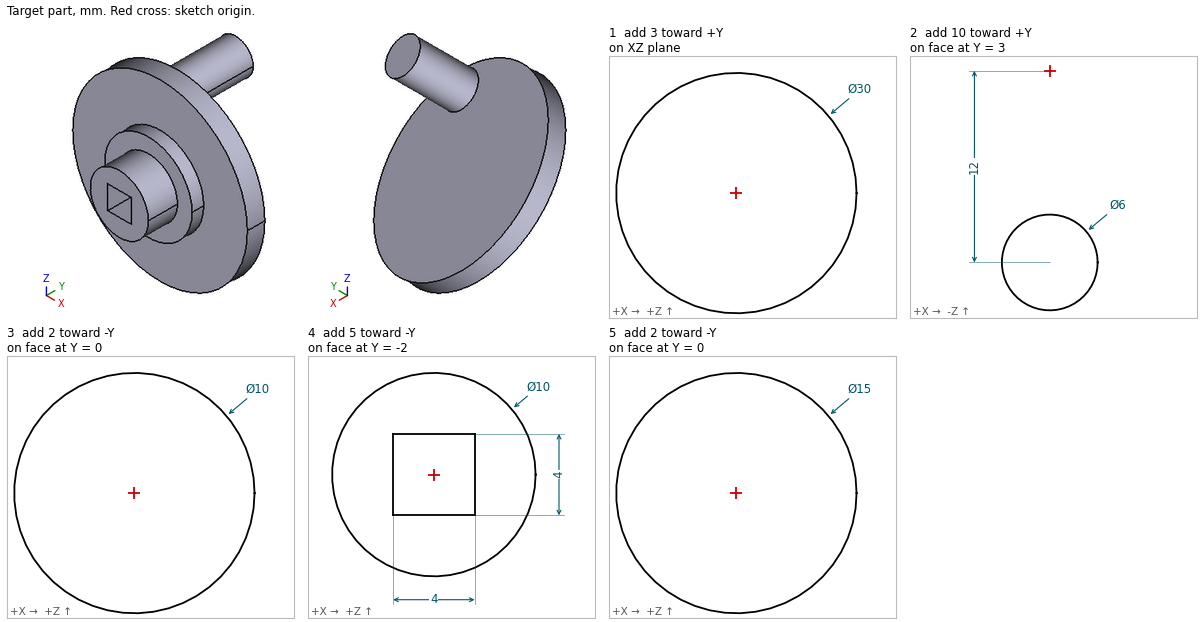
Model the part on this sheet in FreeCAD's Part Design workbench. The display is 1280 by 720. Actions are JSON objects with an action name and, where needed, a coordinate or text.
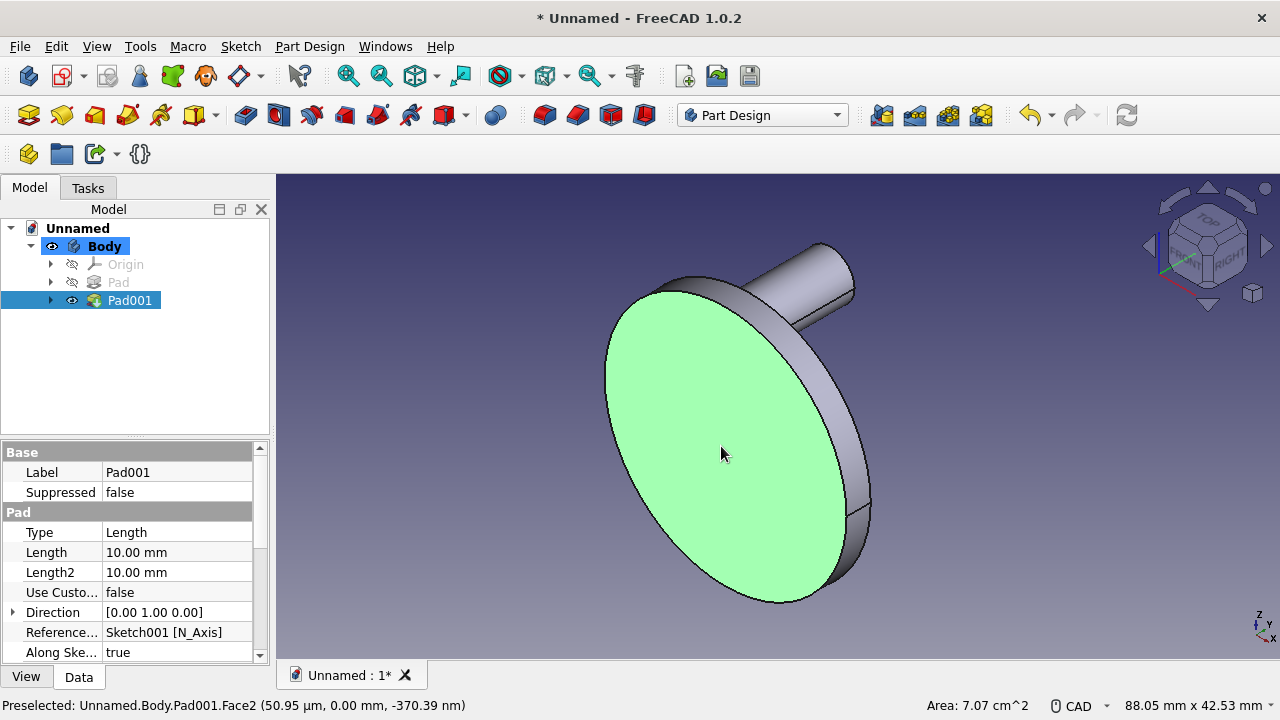
{"action": "left_click", "coordinate": [62, 76]}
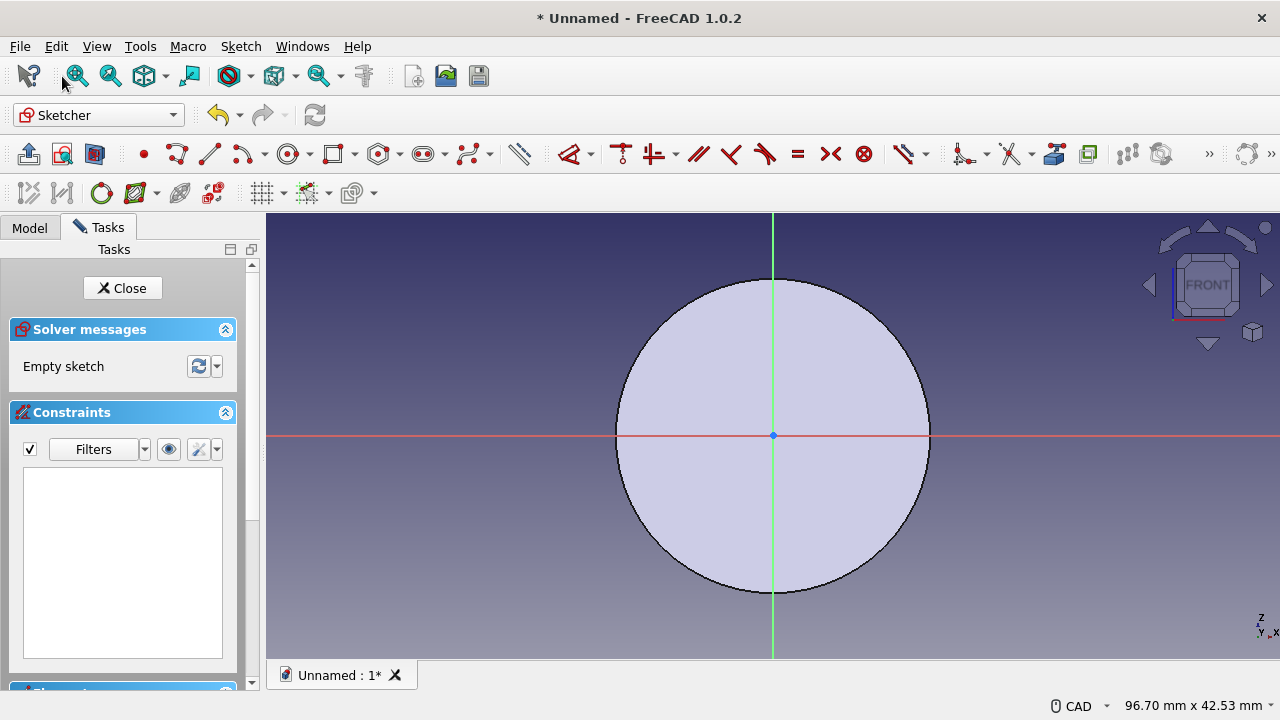
{"action": "scroll", "coordinate": [813, 436], "scroll_direction": "up", "scroll_amount": 5}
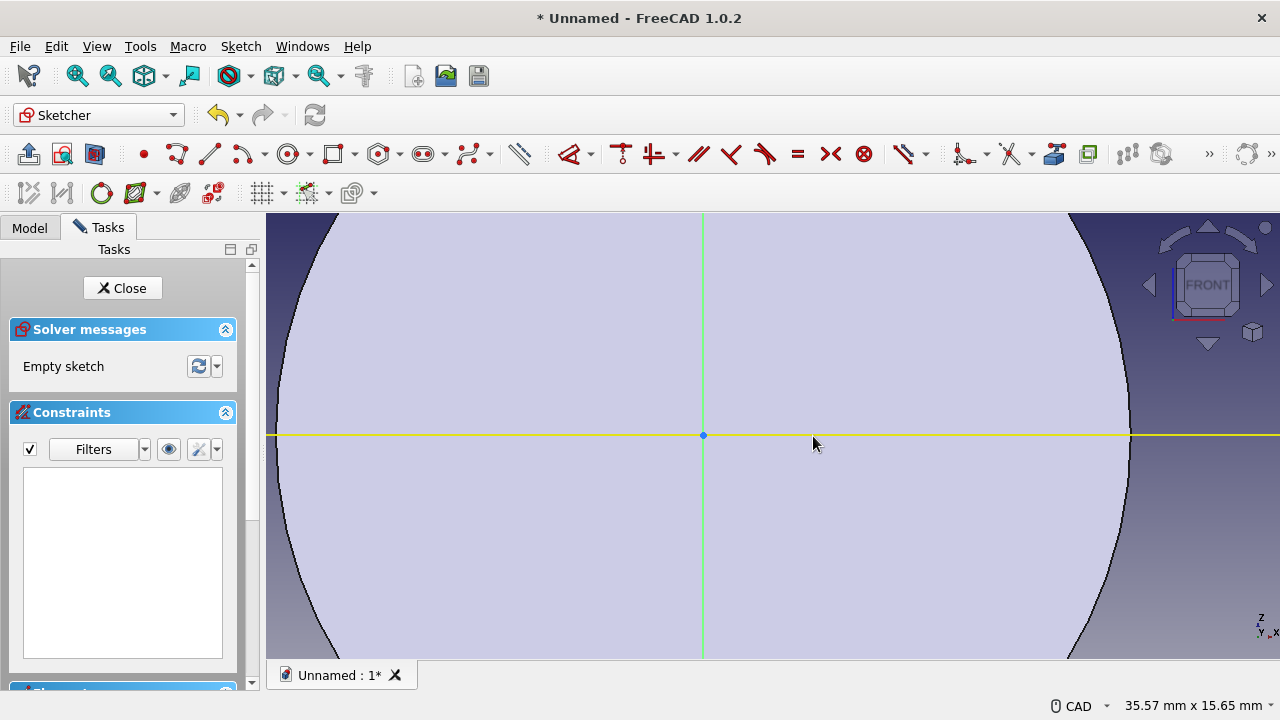
{"action": "left_click", "coordinate": [288, 154]}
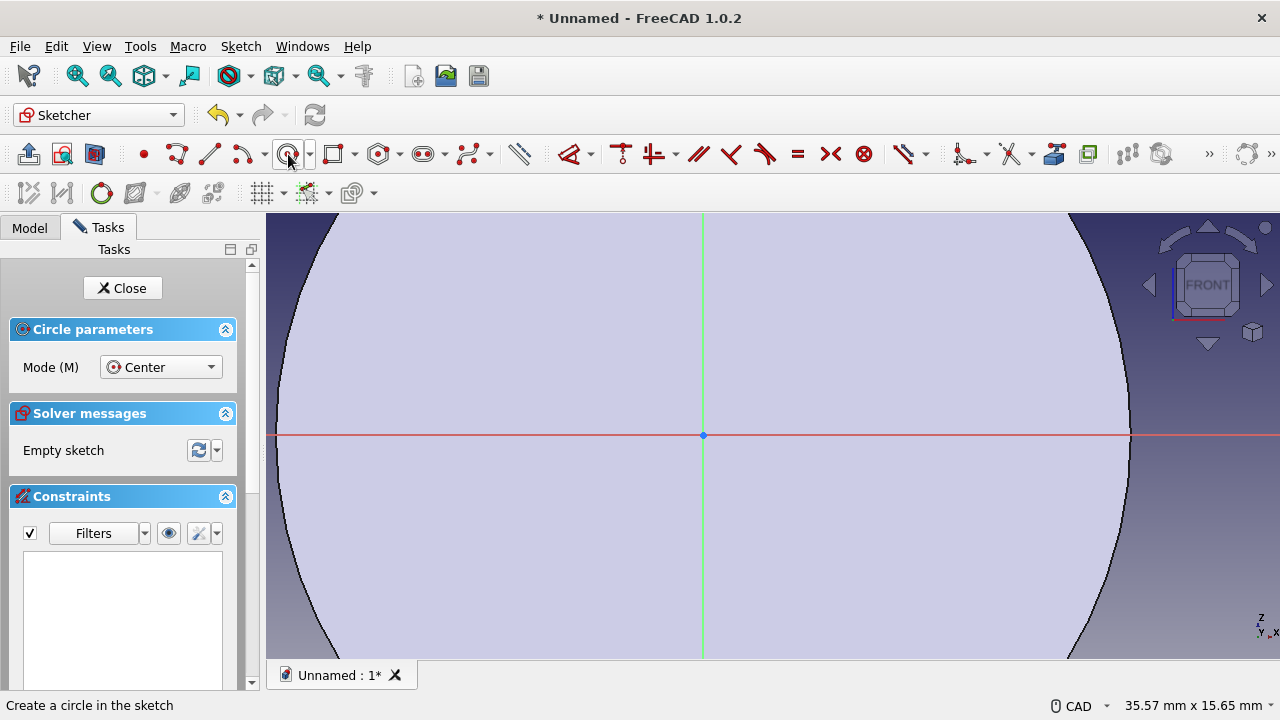
{"action": "left_click", "coordinate": [703, 435]}
{"action": "left_click", "coordinate": [804, 334]}
{"action": "key", "text": "Escape"}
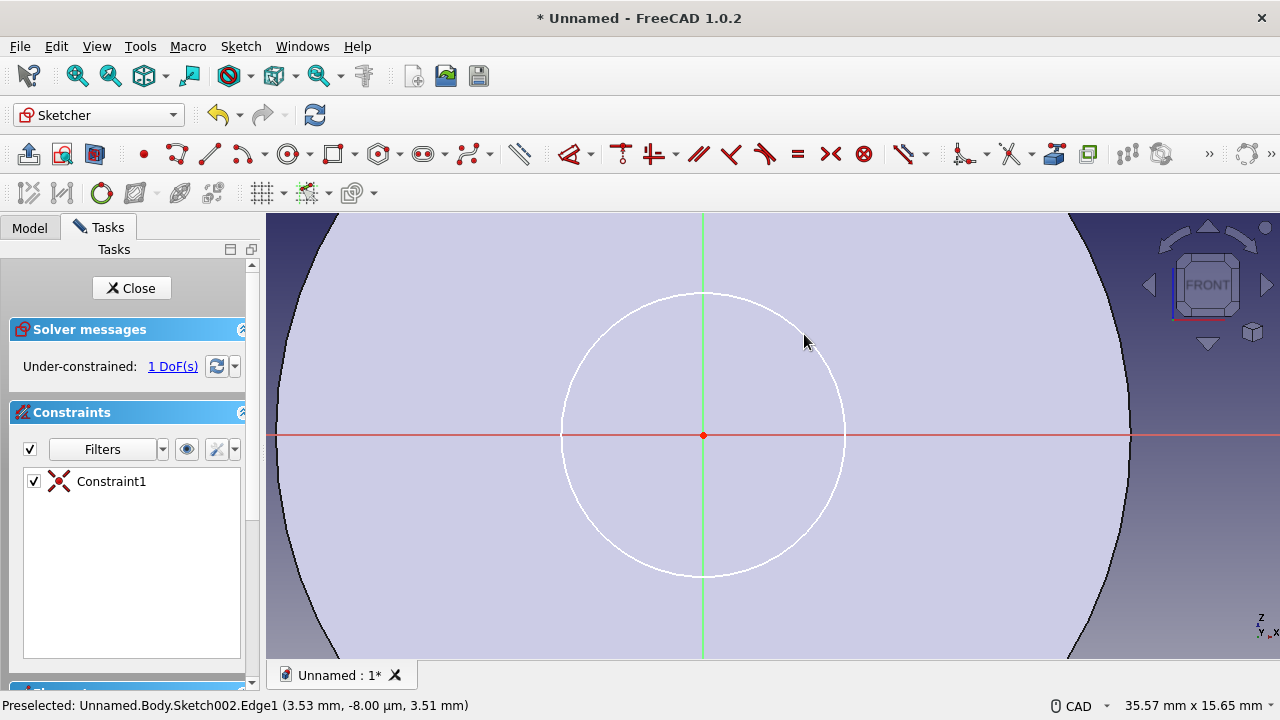
{"action": "left_click", "coordinate": [568, 154]}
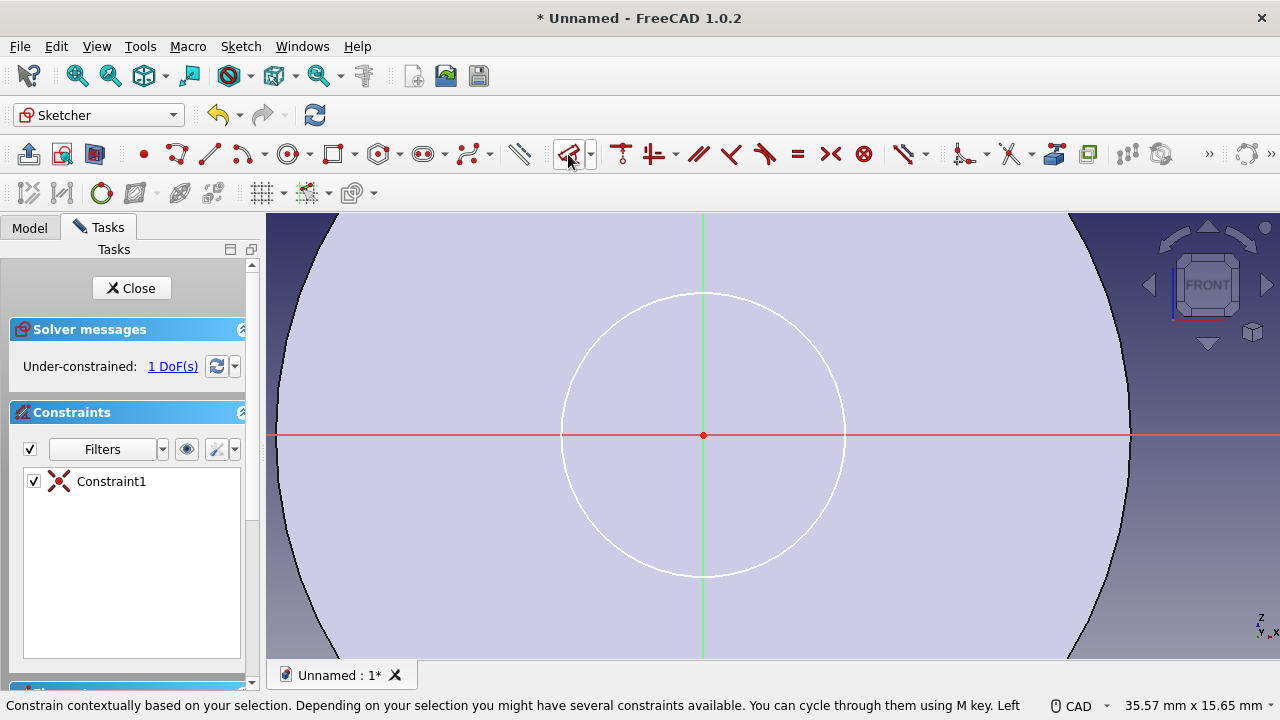
{"action": "left_click", "coordinate": [803, 334]}
{"action": "left_click", "coordinate": [825, 311]}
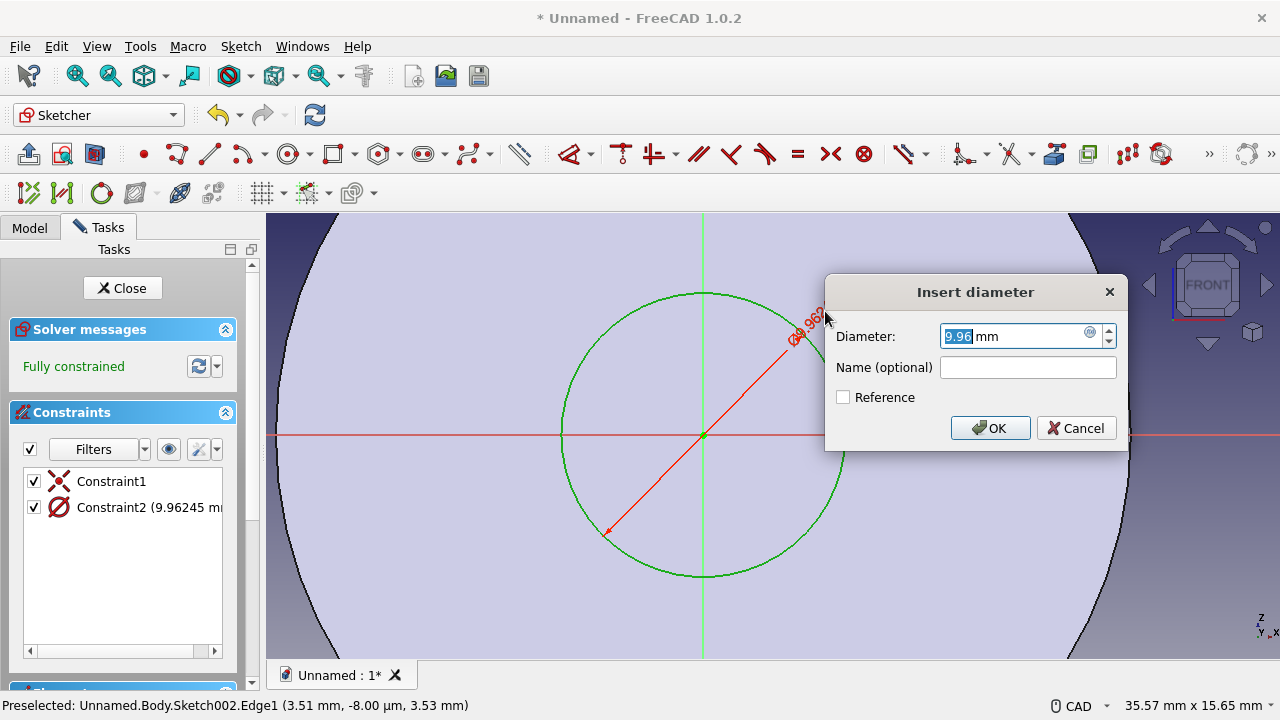
{"action": "type", "text": "10"}
{"action": "key", "text": "Return"}
{"action": "key", "text": "Escape"}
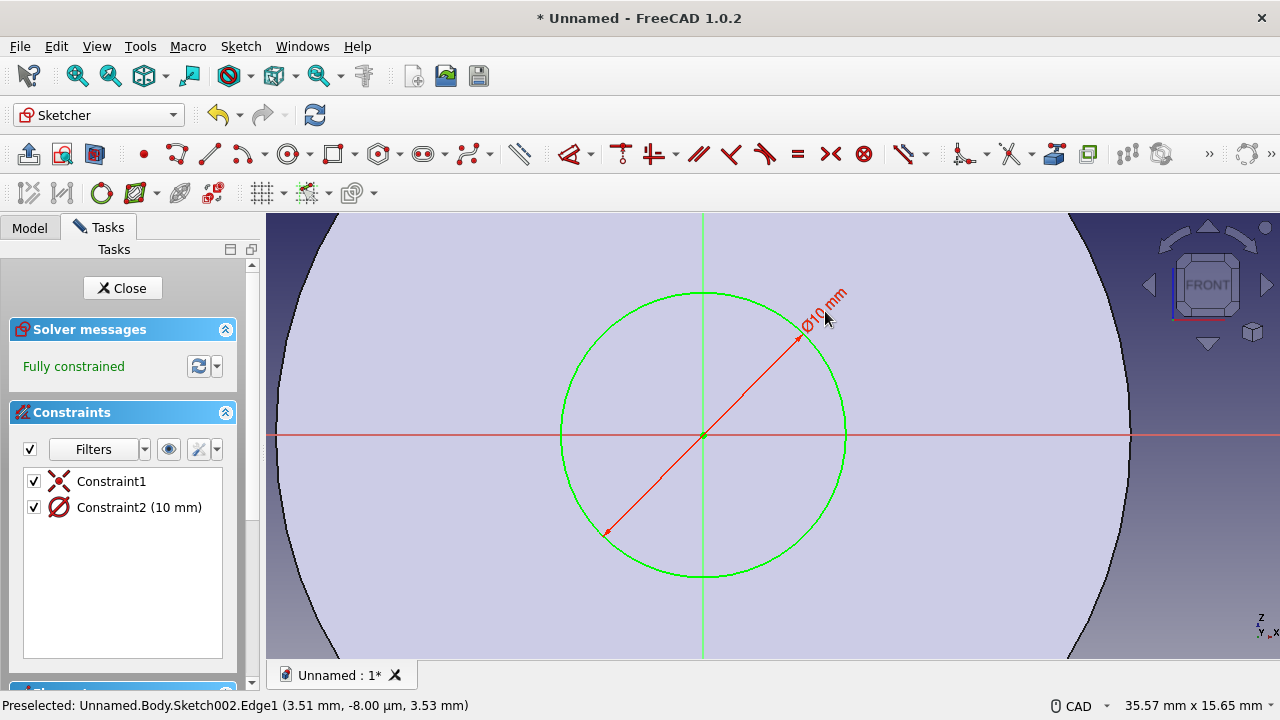
{"action": "left_click", "coordinate": [123, 288]}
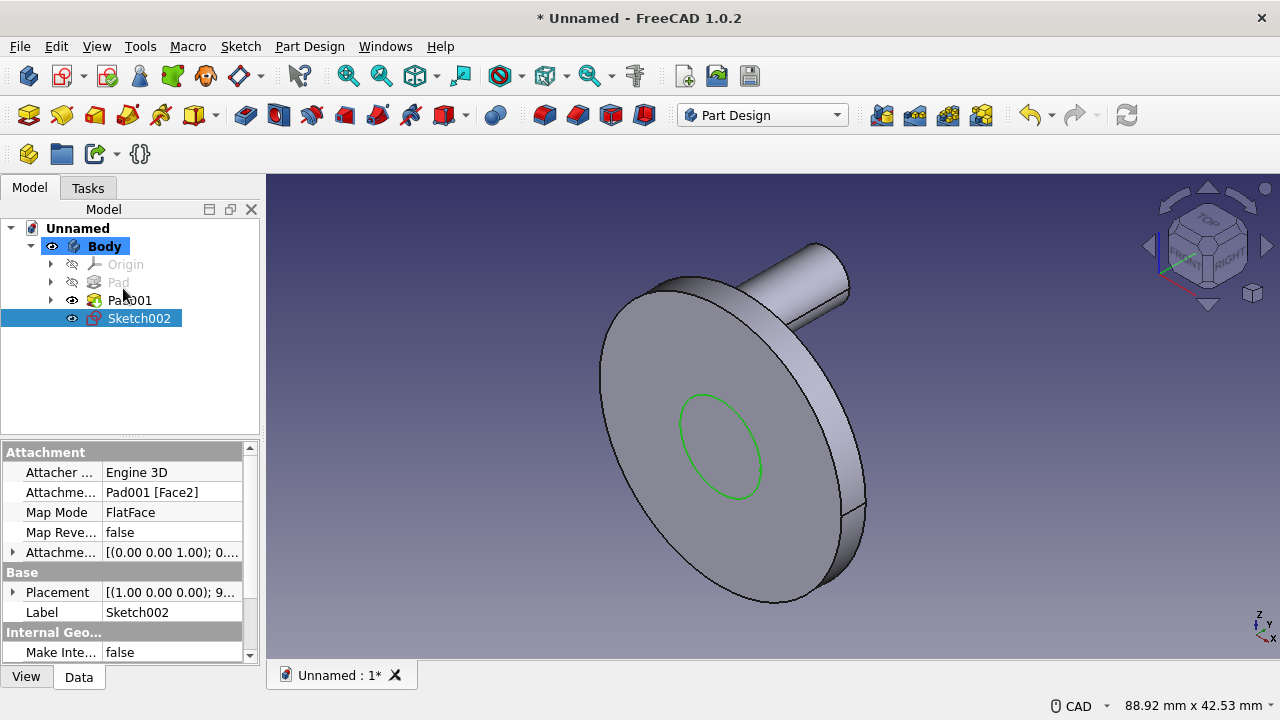
{"action": "left_click", "coordinate": [29, 116]}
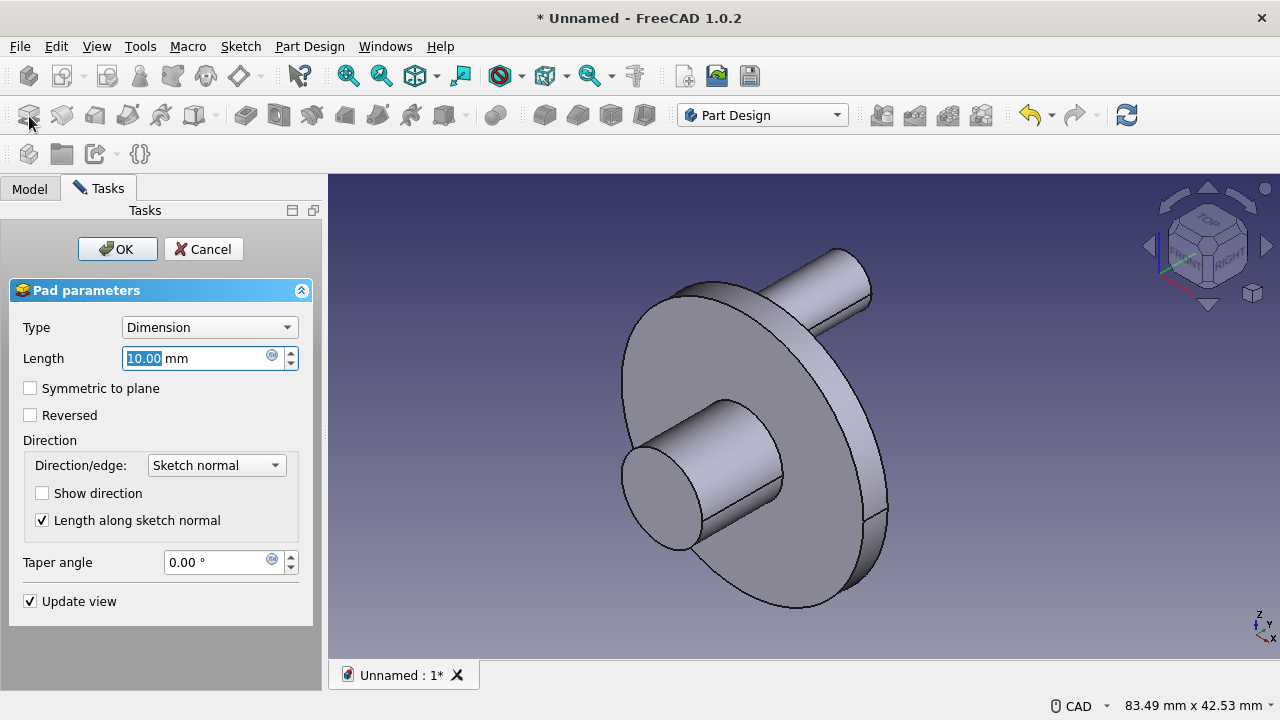
{"action": "type", "text": "2"}
{"action": "key", "text": "Tab"}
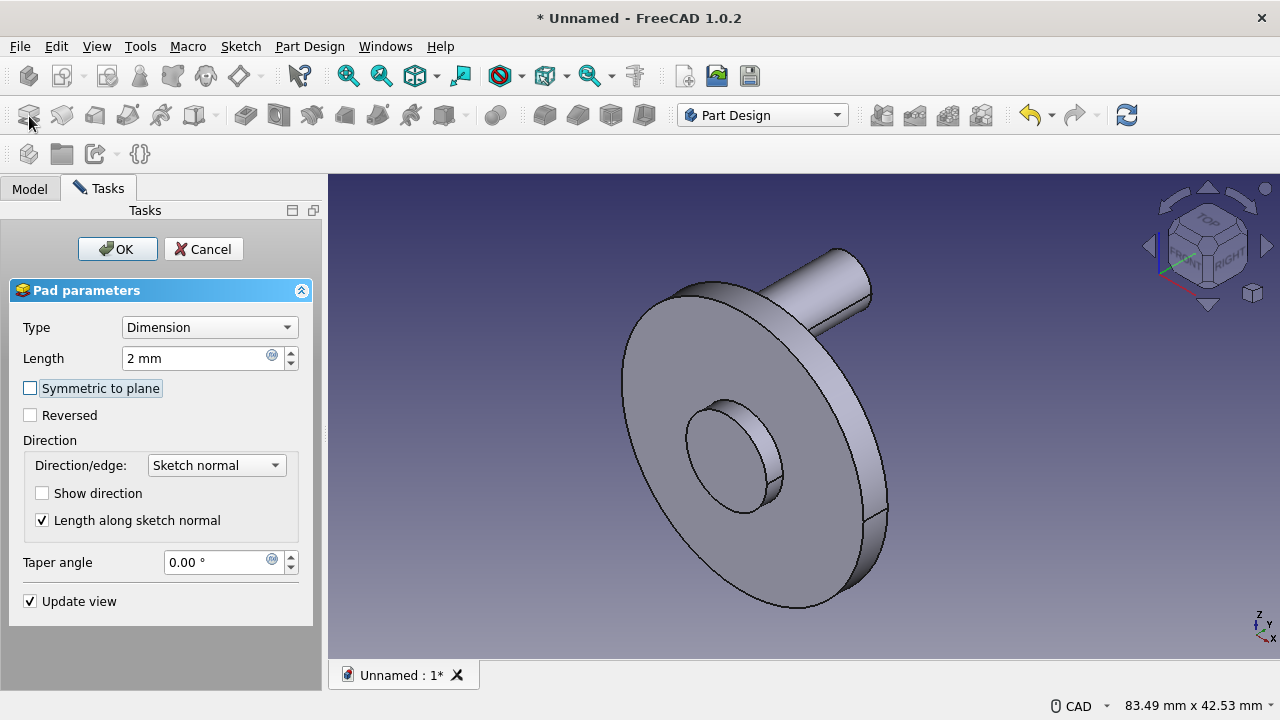
{"action": "left_click", "coordinate": [118, 249]}